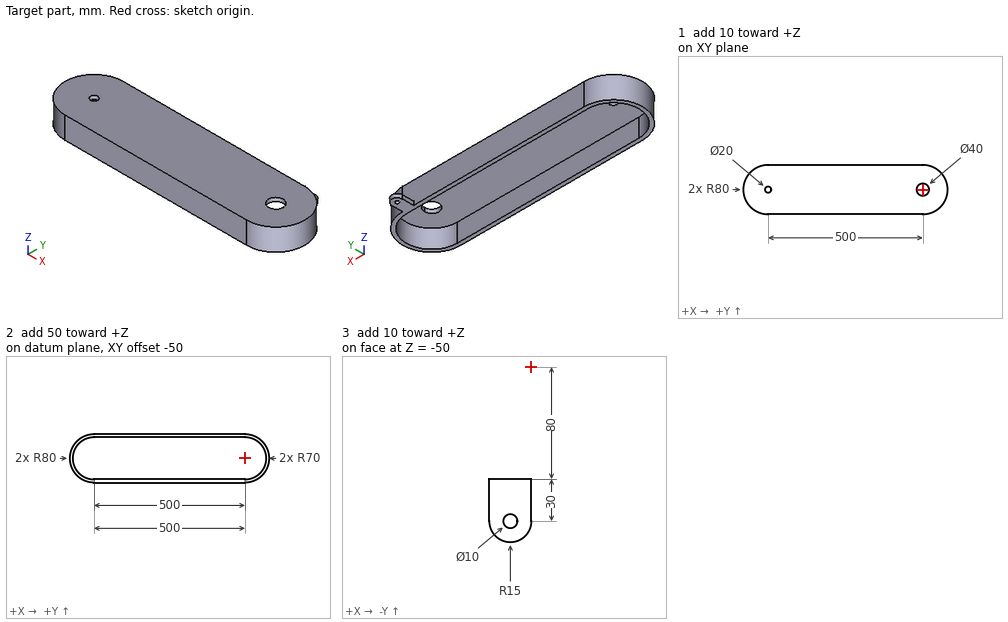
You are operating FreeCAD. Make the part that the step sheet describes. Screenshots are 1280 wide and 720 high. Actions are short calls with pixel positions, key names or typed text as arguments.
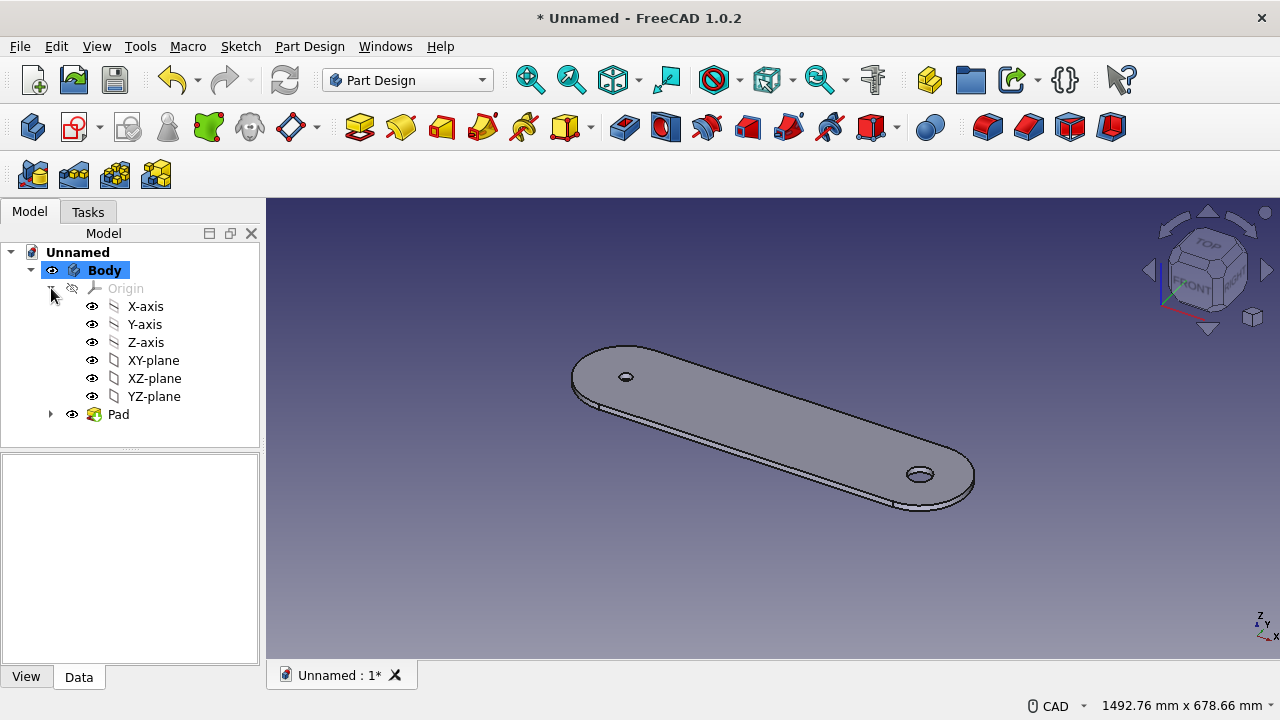
click(137, 360)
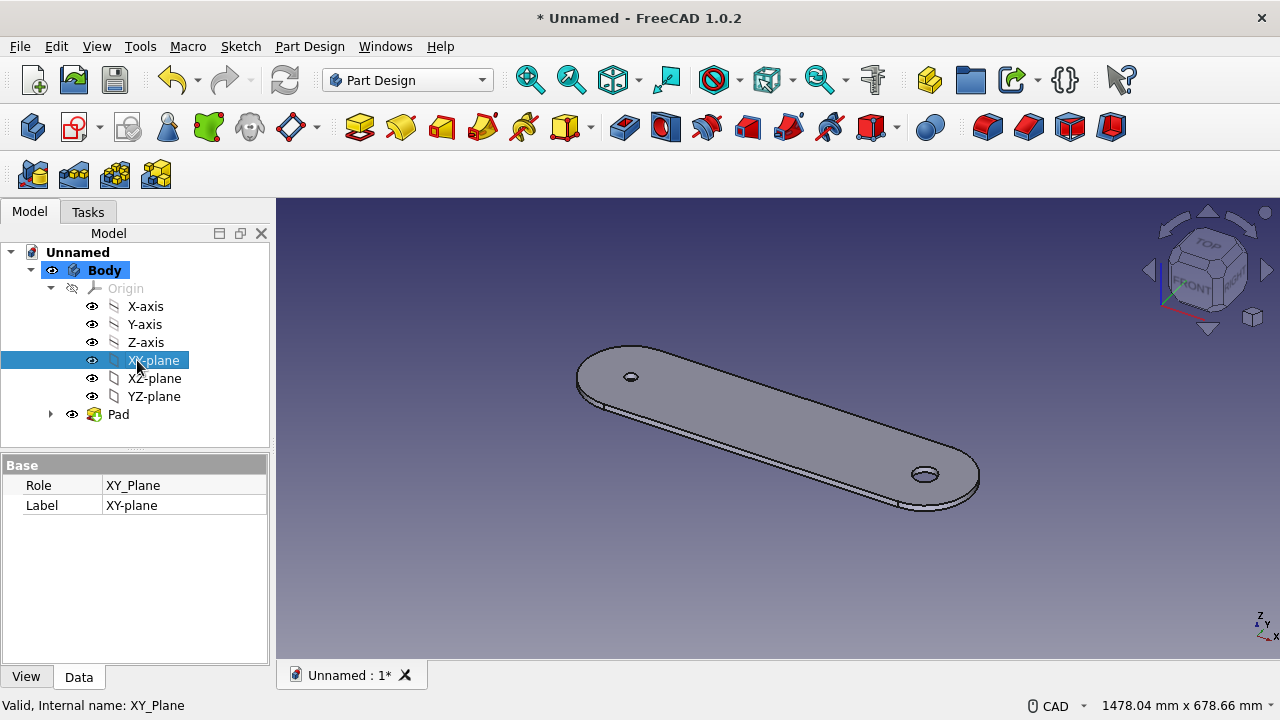
click(290, 128)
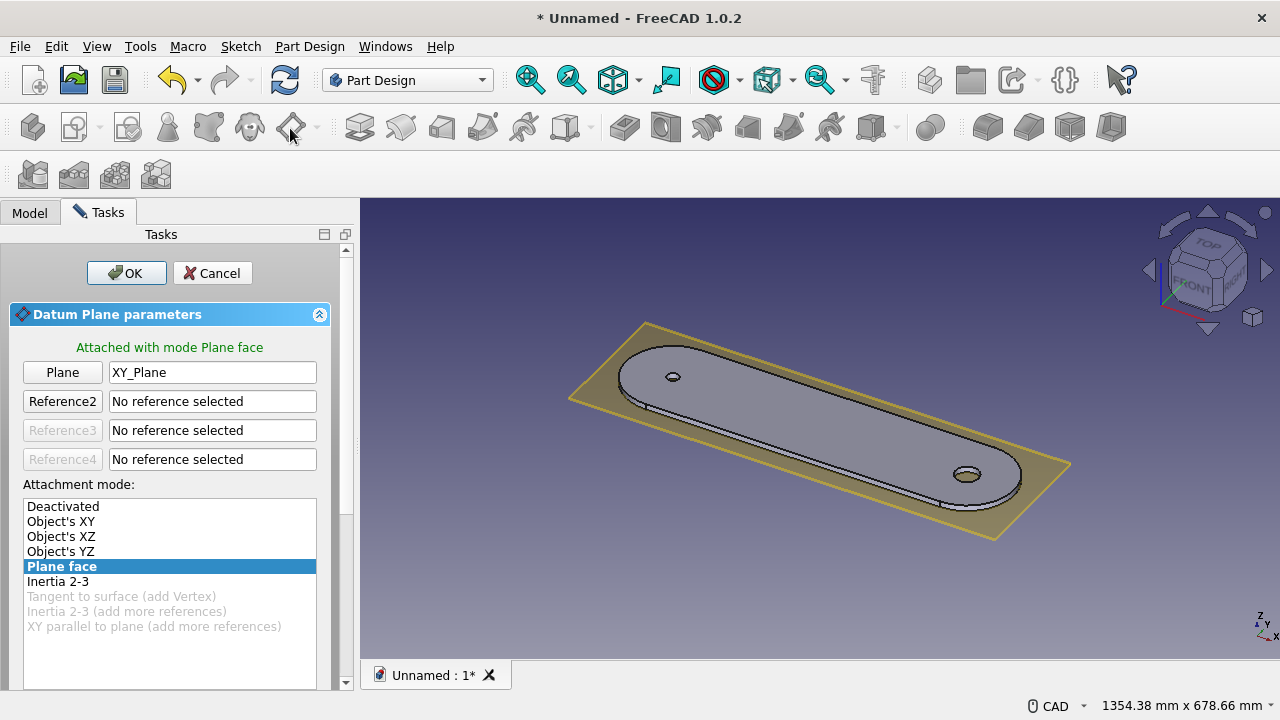
scroll(346, 467, down, 4)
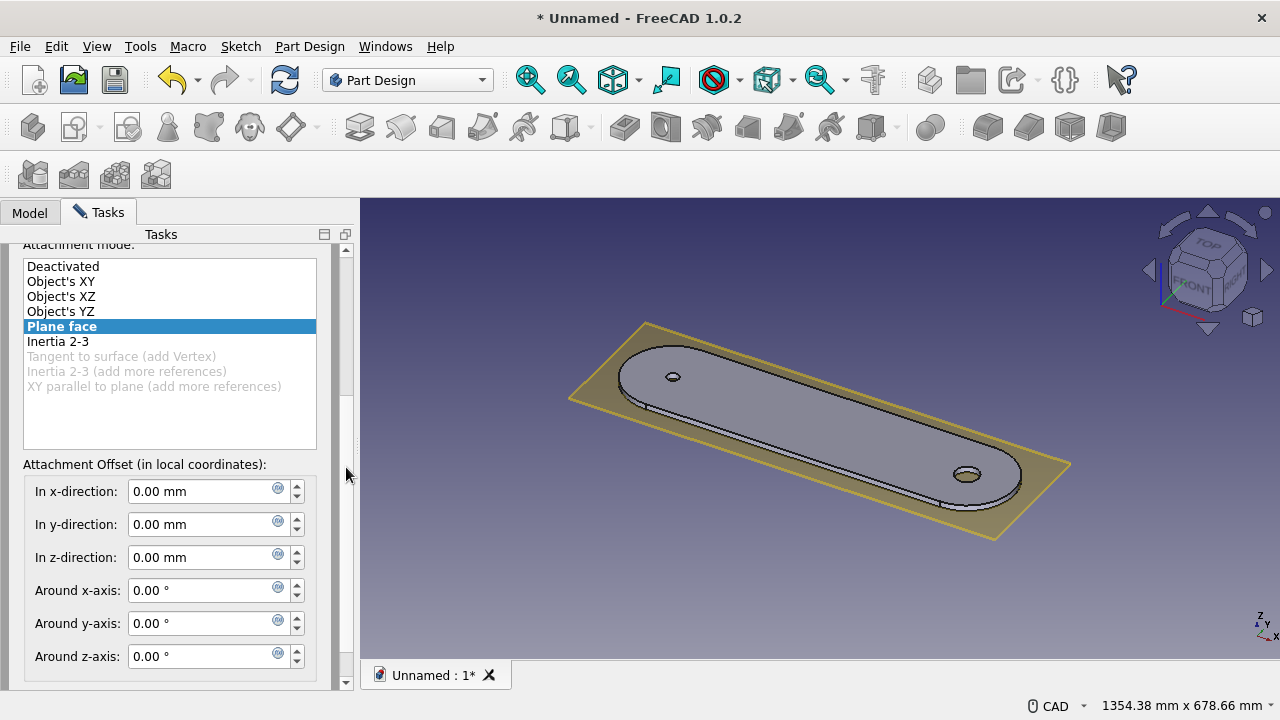
triple_click(210, 558)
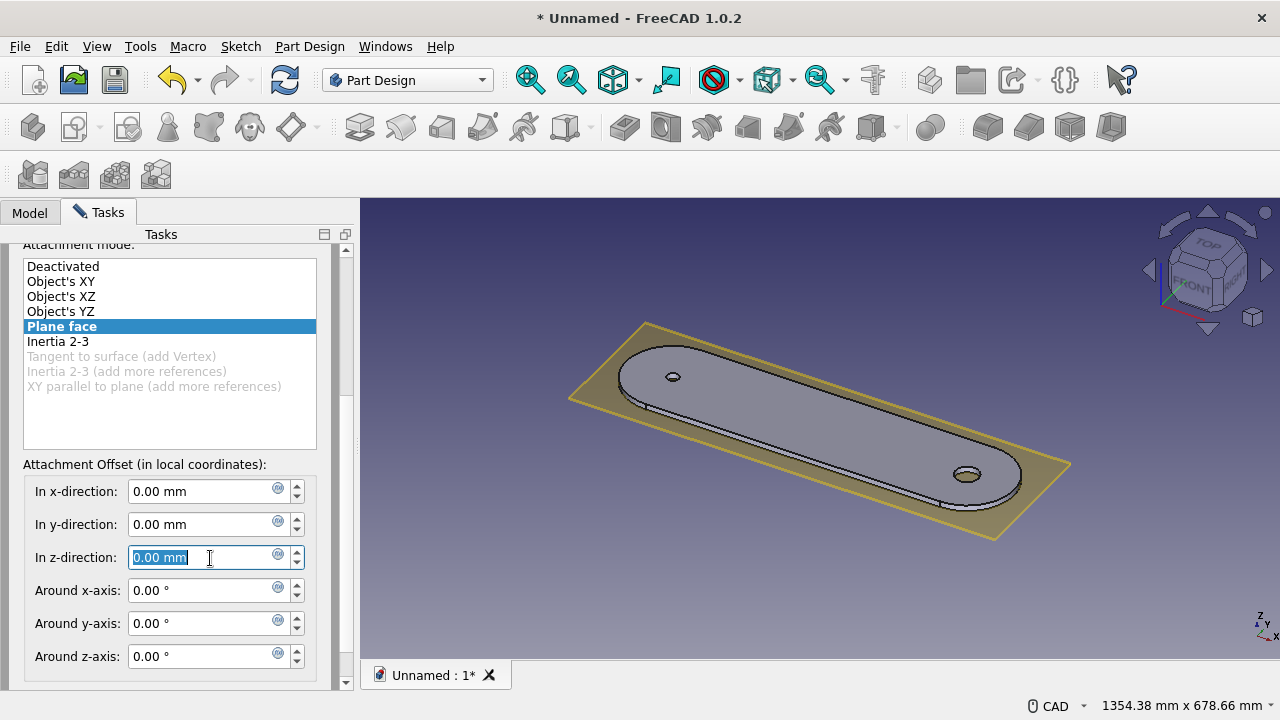
text(-50)
key(Tab)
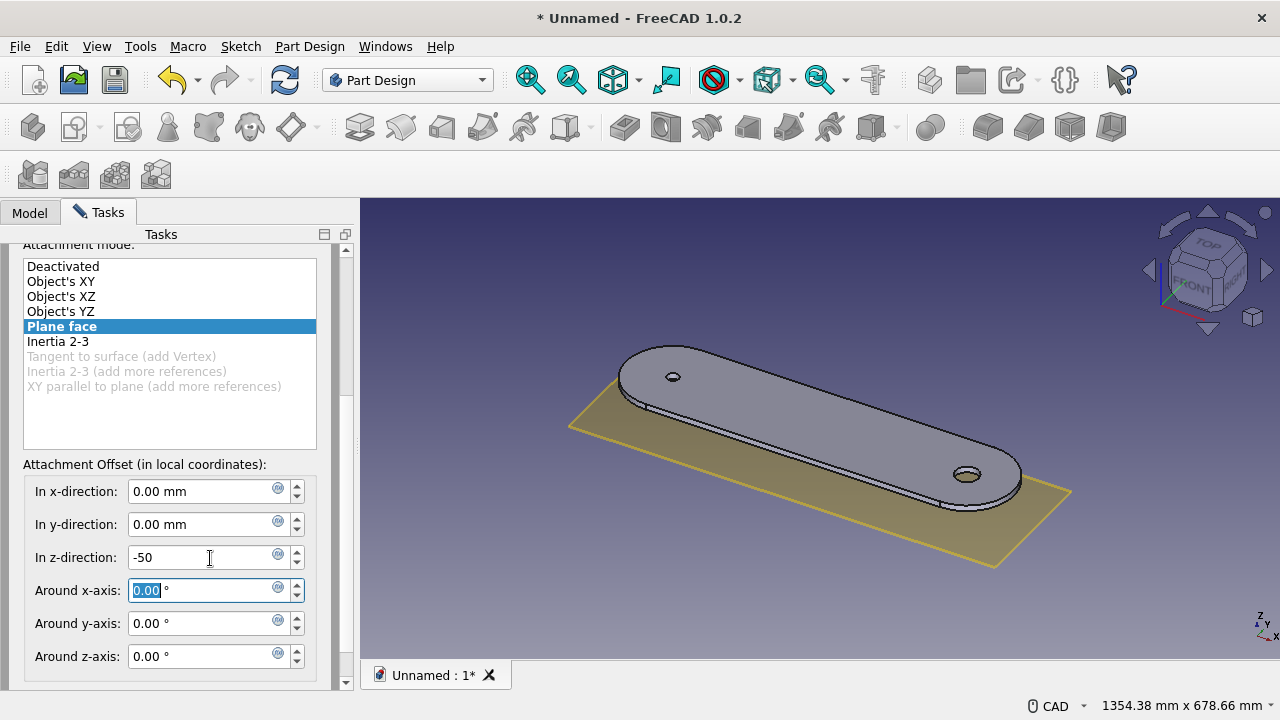
scroll(346, 467, up, 5)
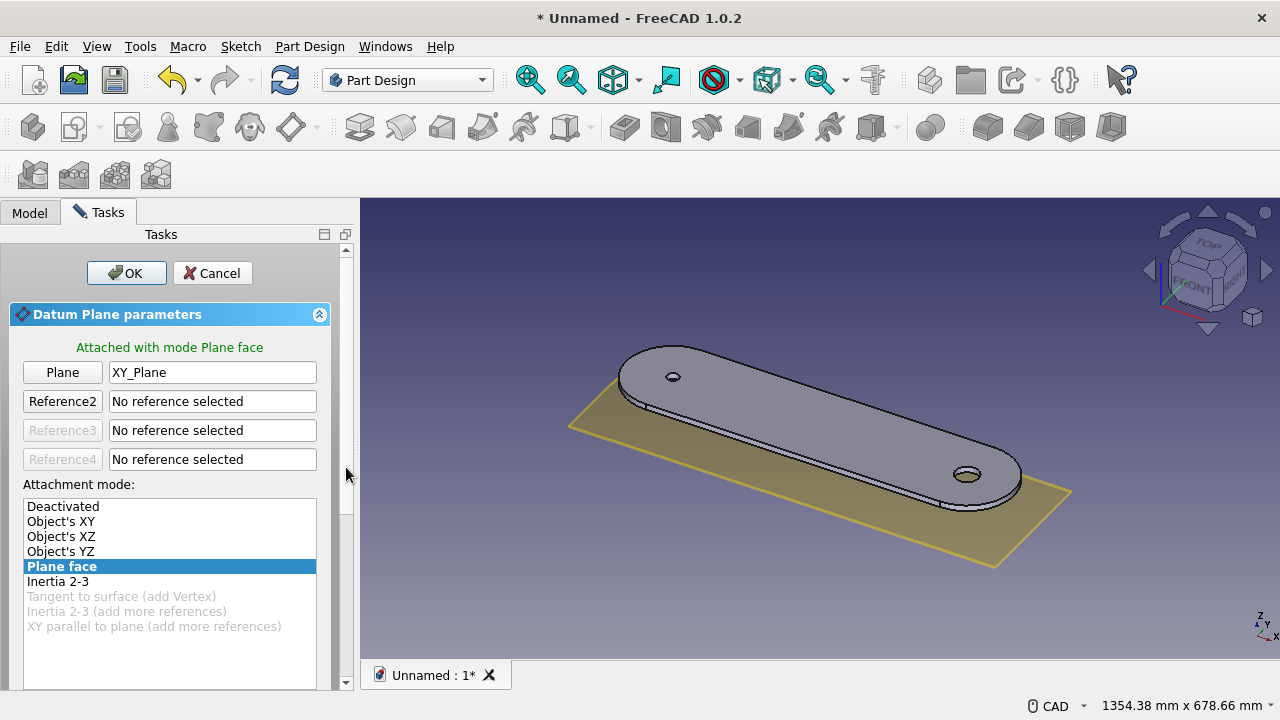
click(127, 273)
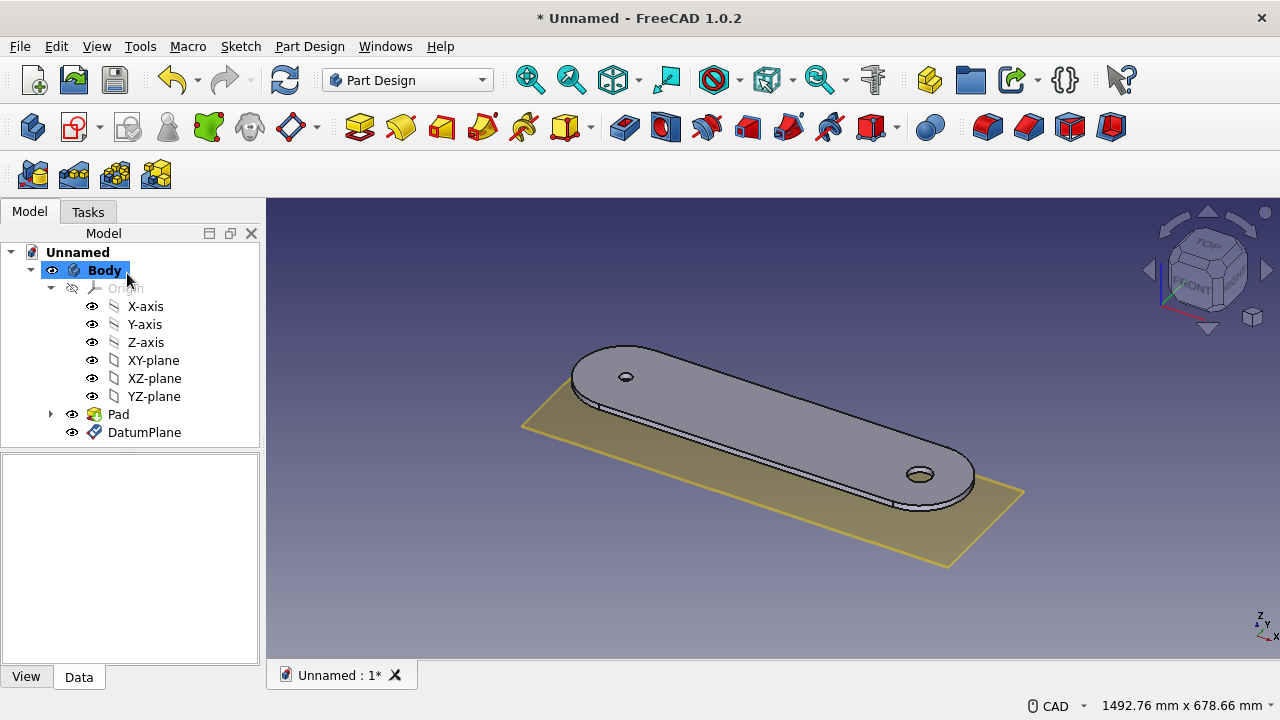
click(117, 432)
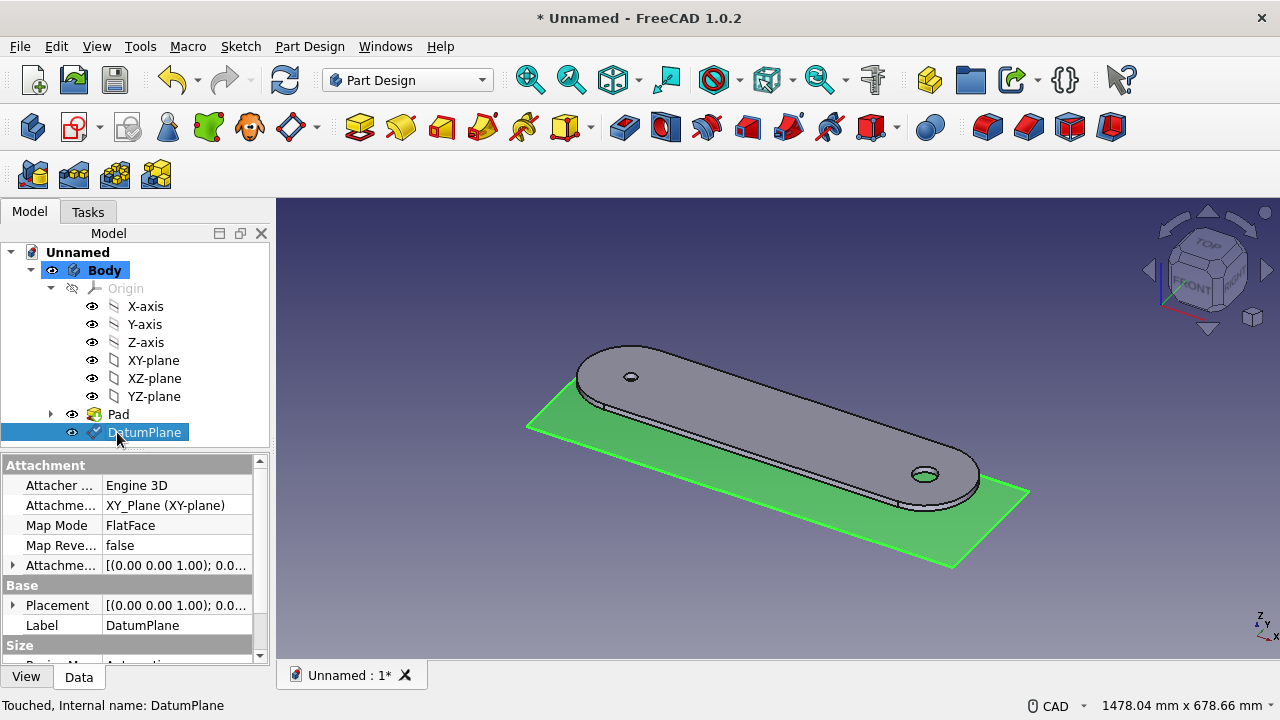
click(74, 128)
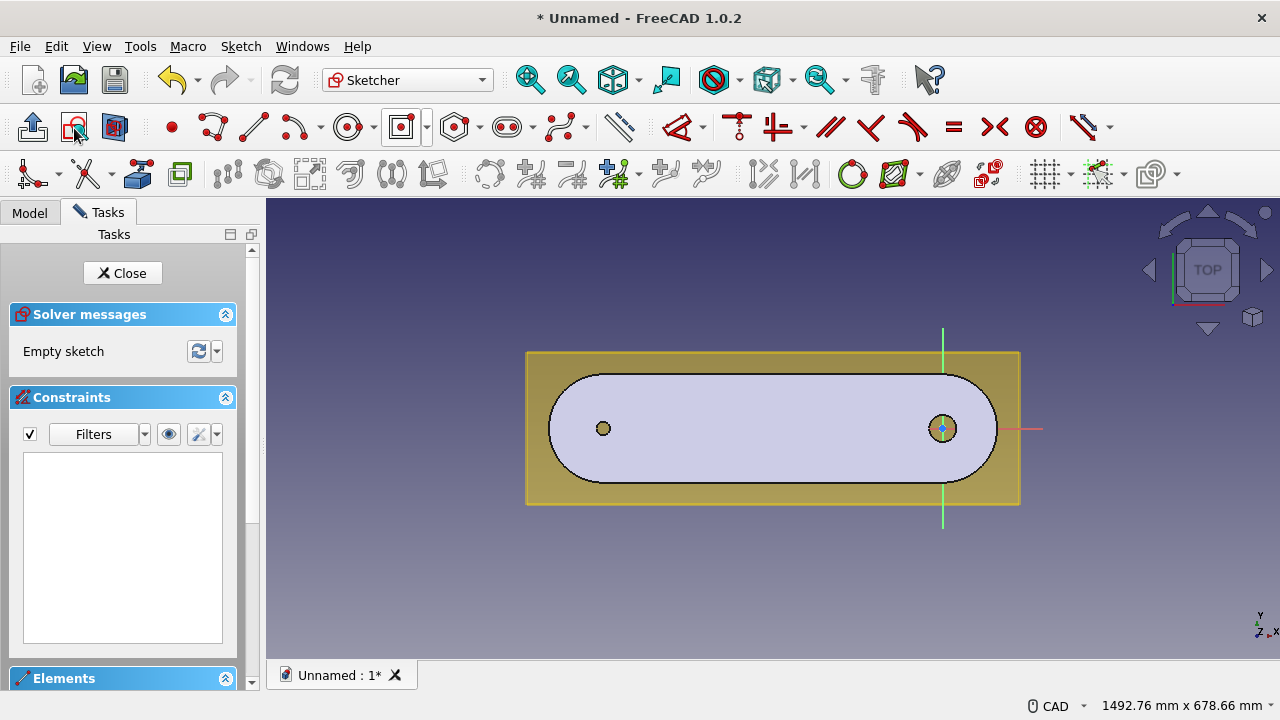
click(115, 128)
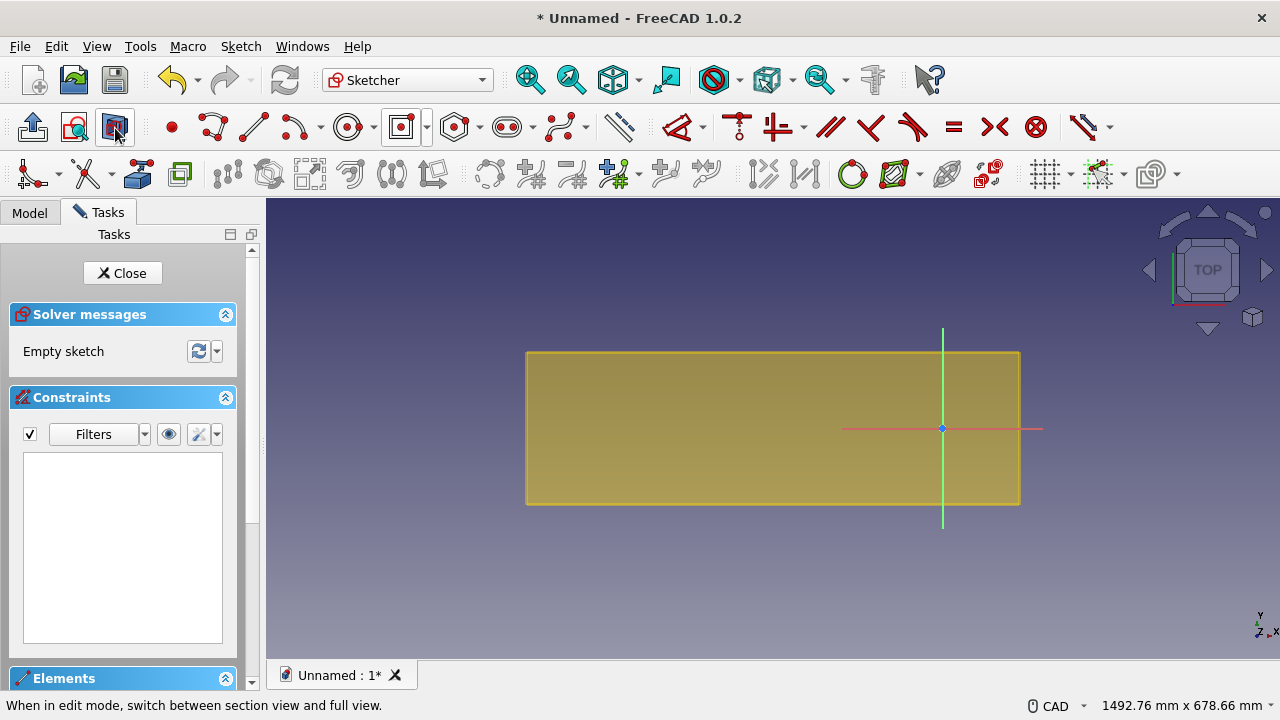
click(506, 128)